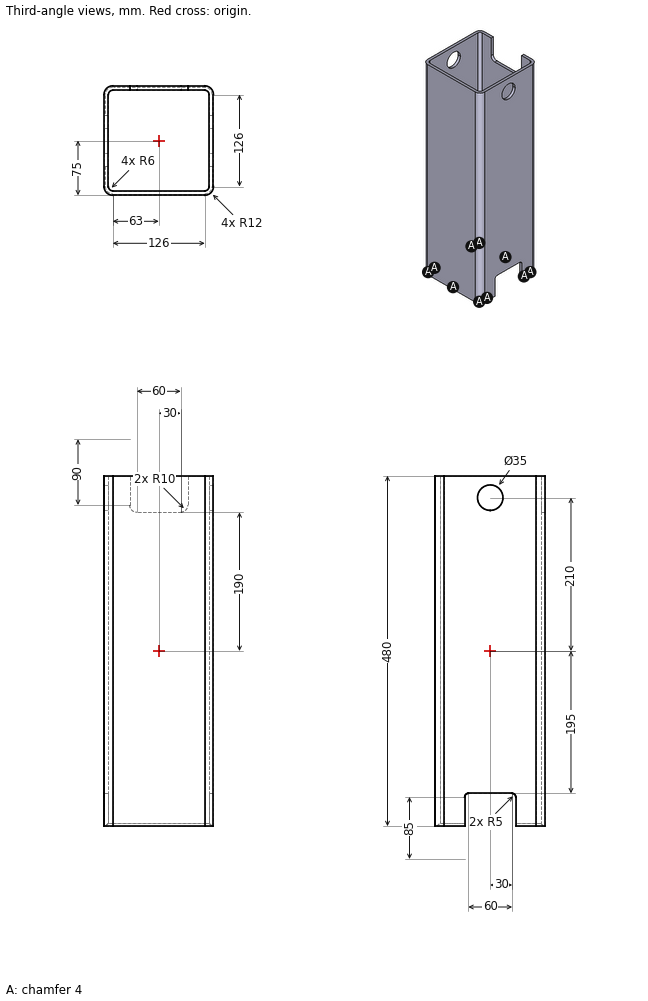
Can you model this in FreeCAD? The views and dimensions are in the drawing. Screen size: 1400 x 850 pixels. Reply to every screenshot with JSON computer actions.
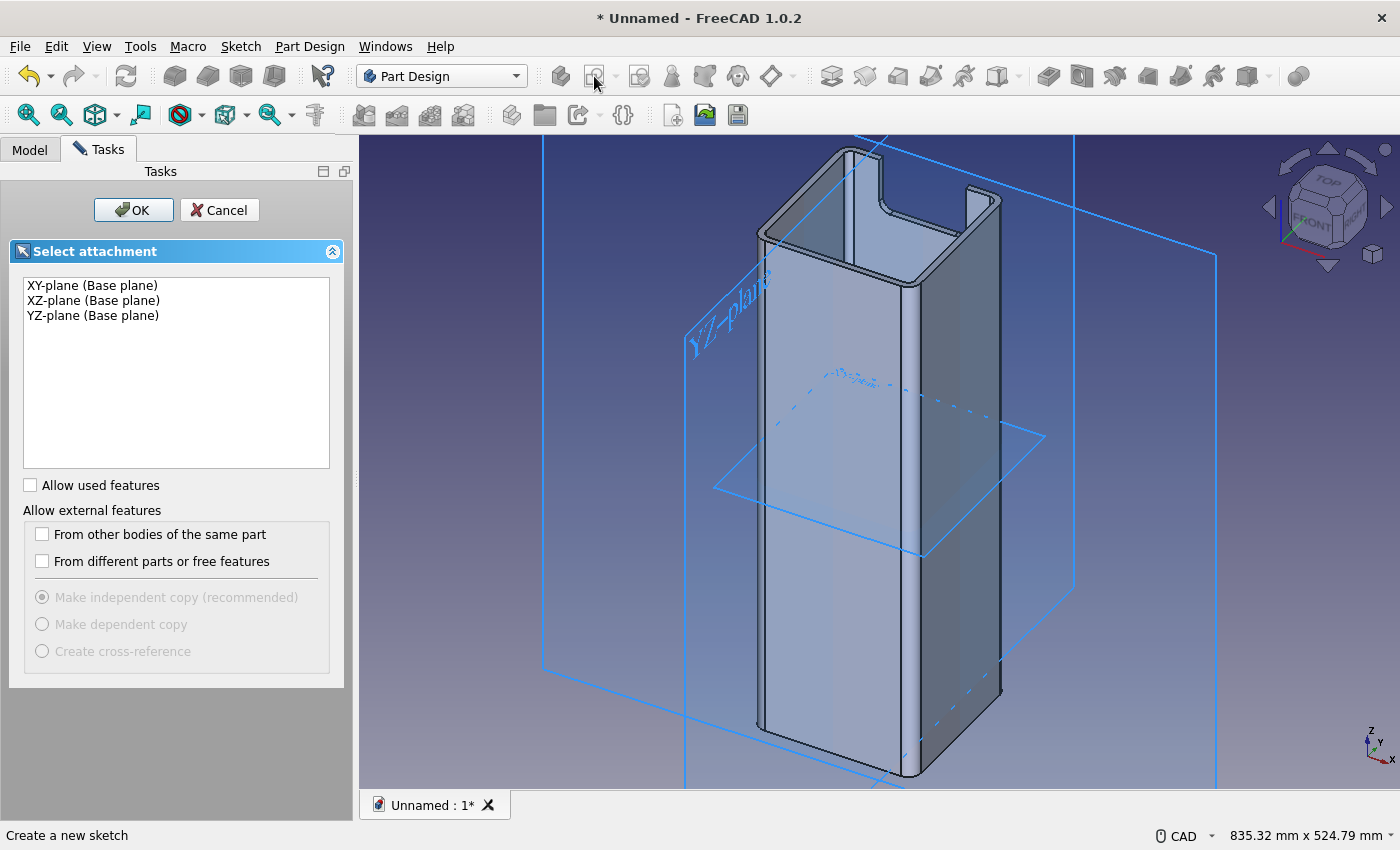
{"action": "left_click", "coordinate": [84, 316]}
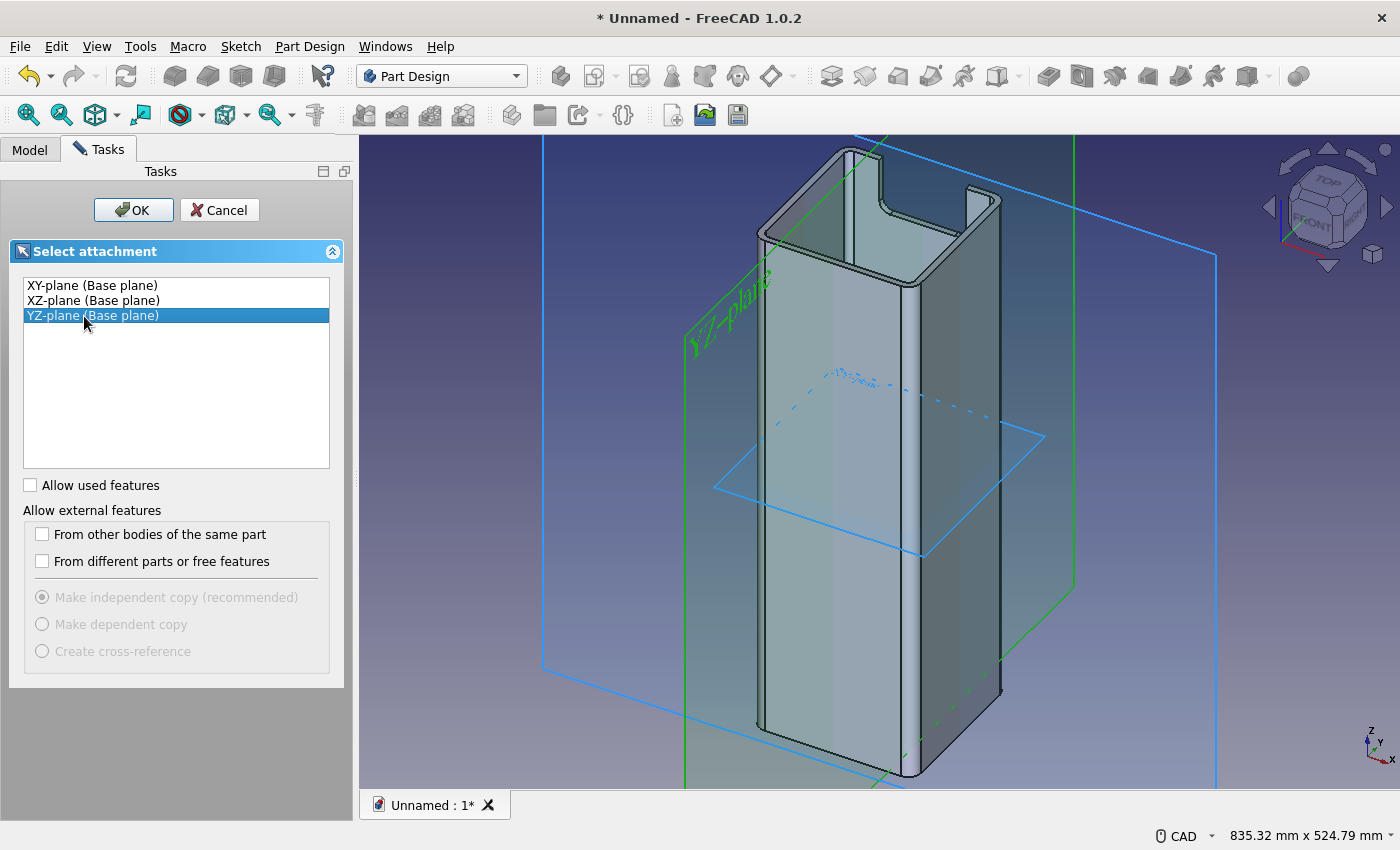
{"action": "left_click", "coordinate": [134, 210]}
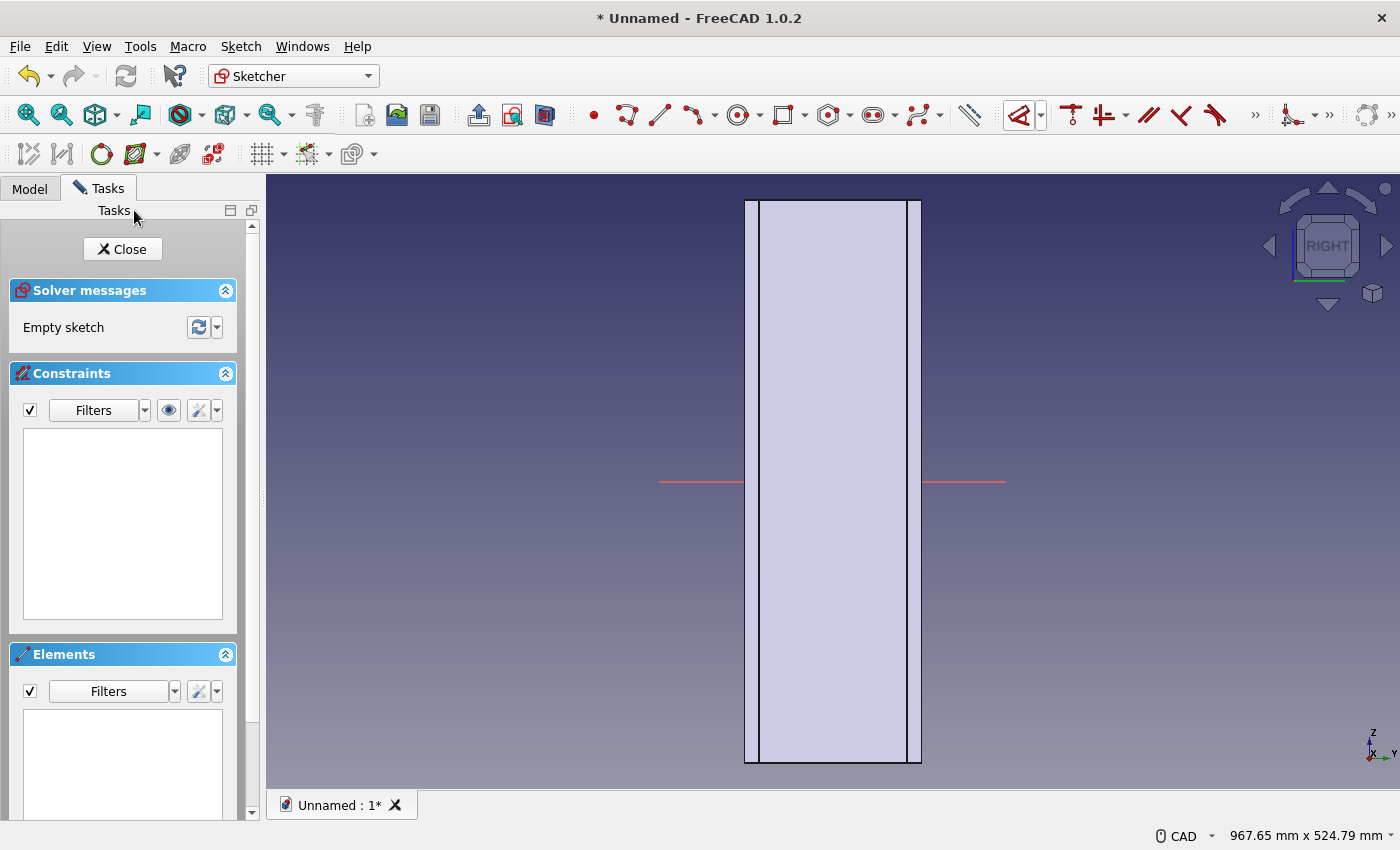
{"action": "left_click", "coordinate": [545, 116]}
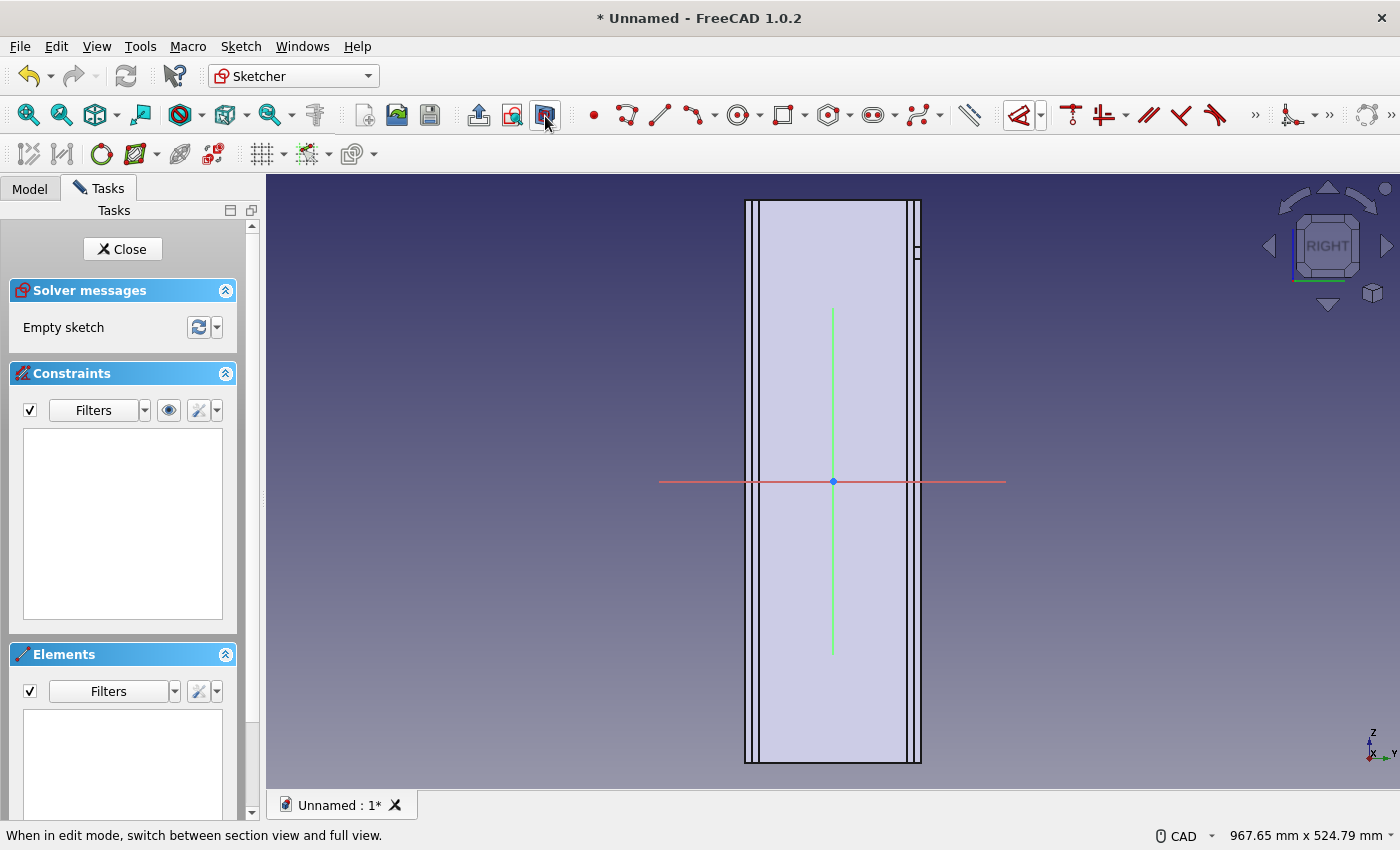
{"action": "scroll", "coordinate": [625, 413], "scroll_direction": "down", "scroll_amount": 2}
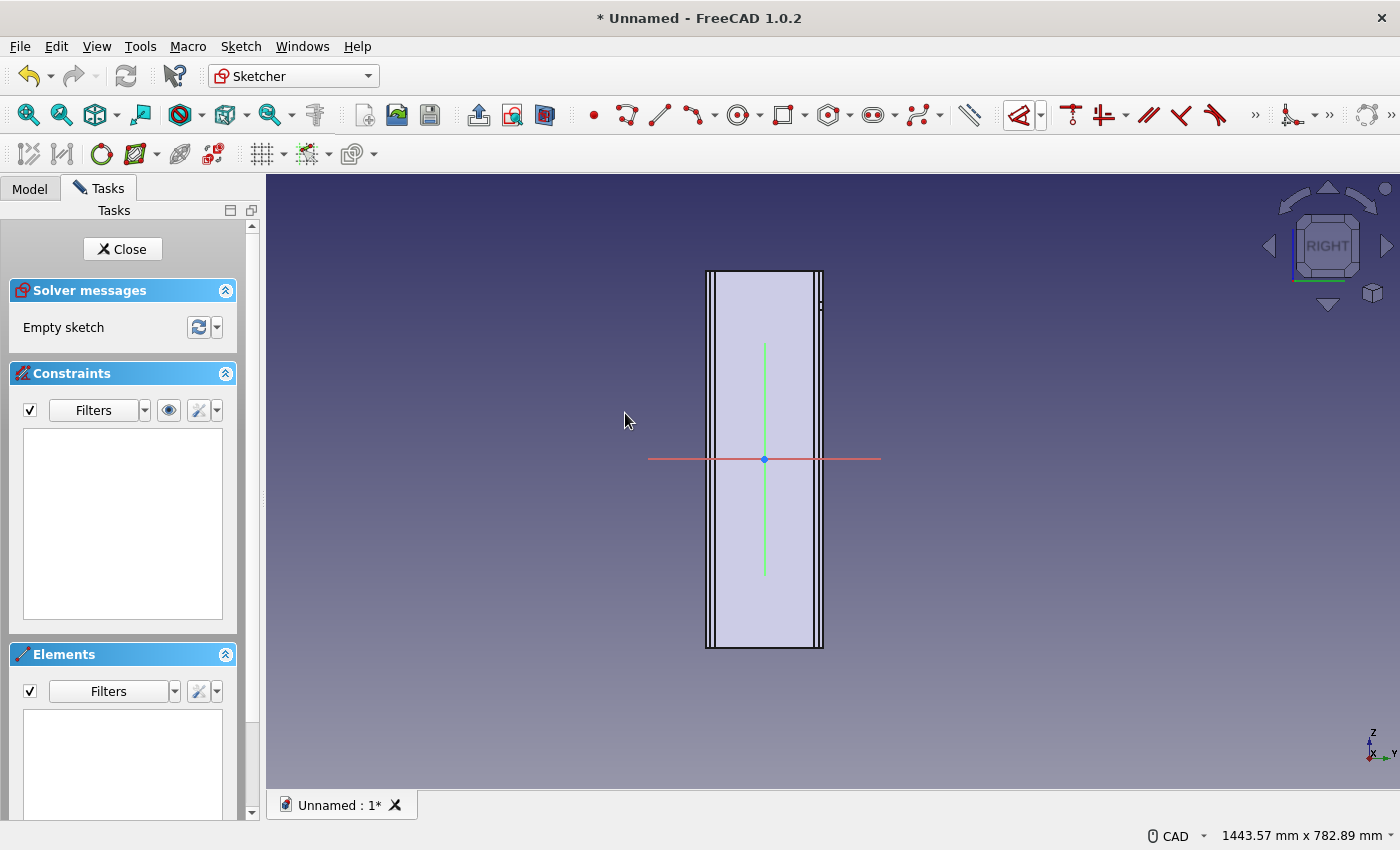
{"action": "left_click", "coordinate": [660, 116]}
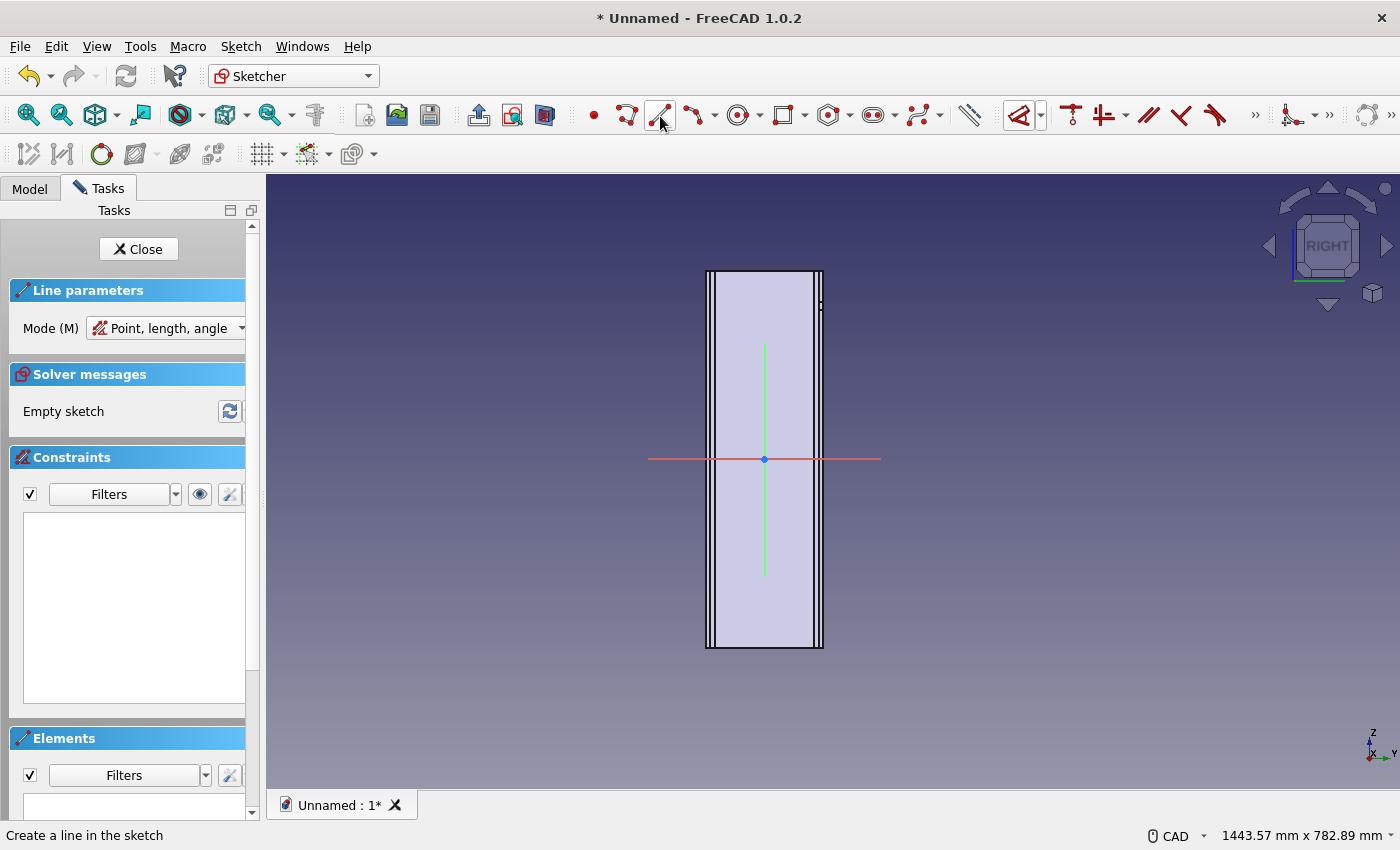
{"action": "left_click", "coordinate": [788, 612]}
{"action": "left_click", "coordinate": [741, 612]}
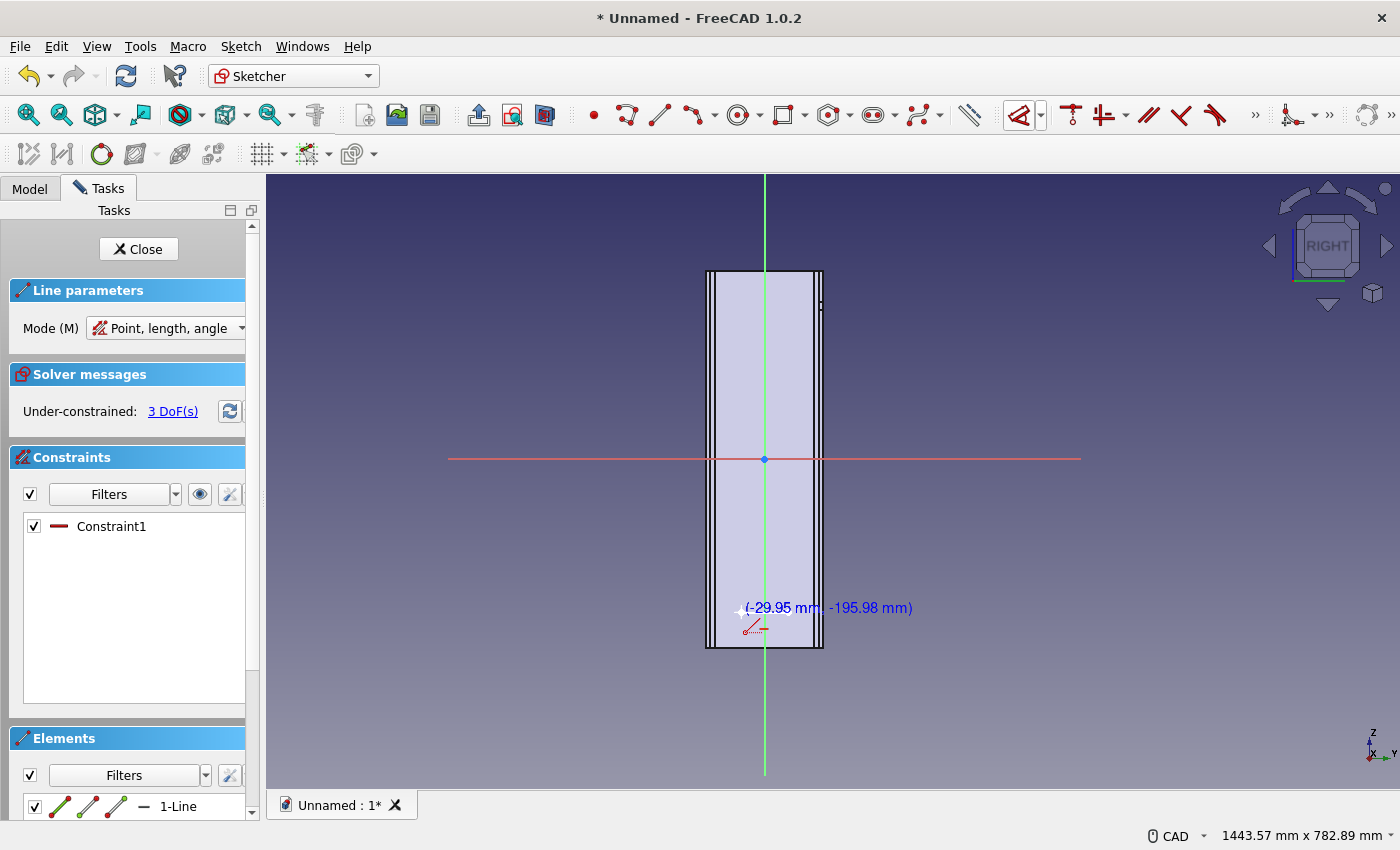
{"action": "left_click", "coordinate": [627, 116]}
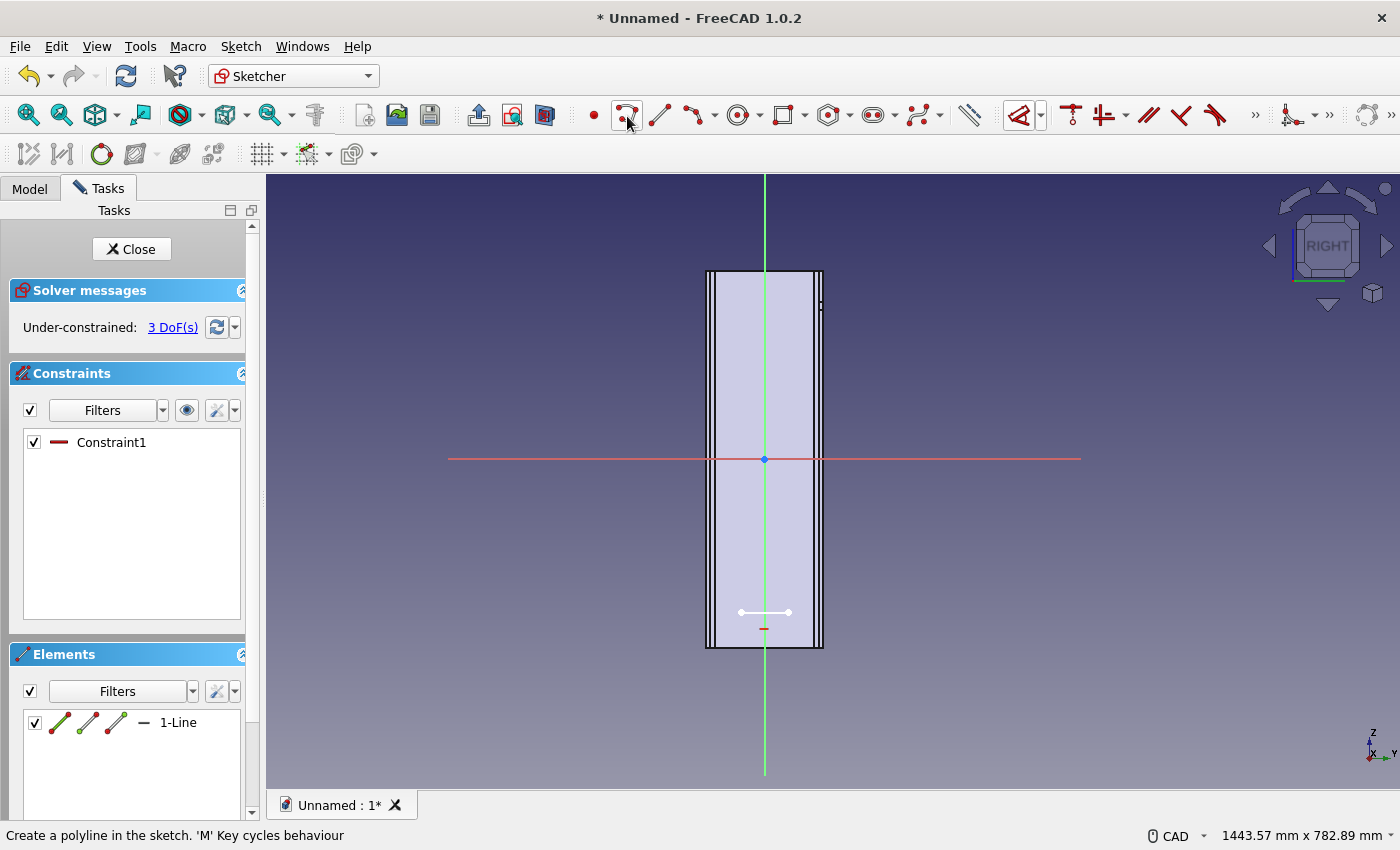
{"action": "scroll", "coordinate": [737, 616], "scroll_direction": "up", "scroll_amount": 6}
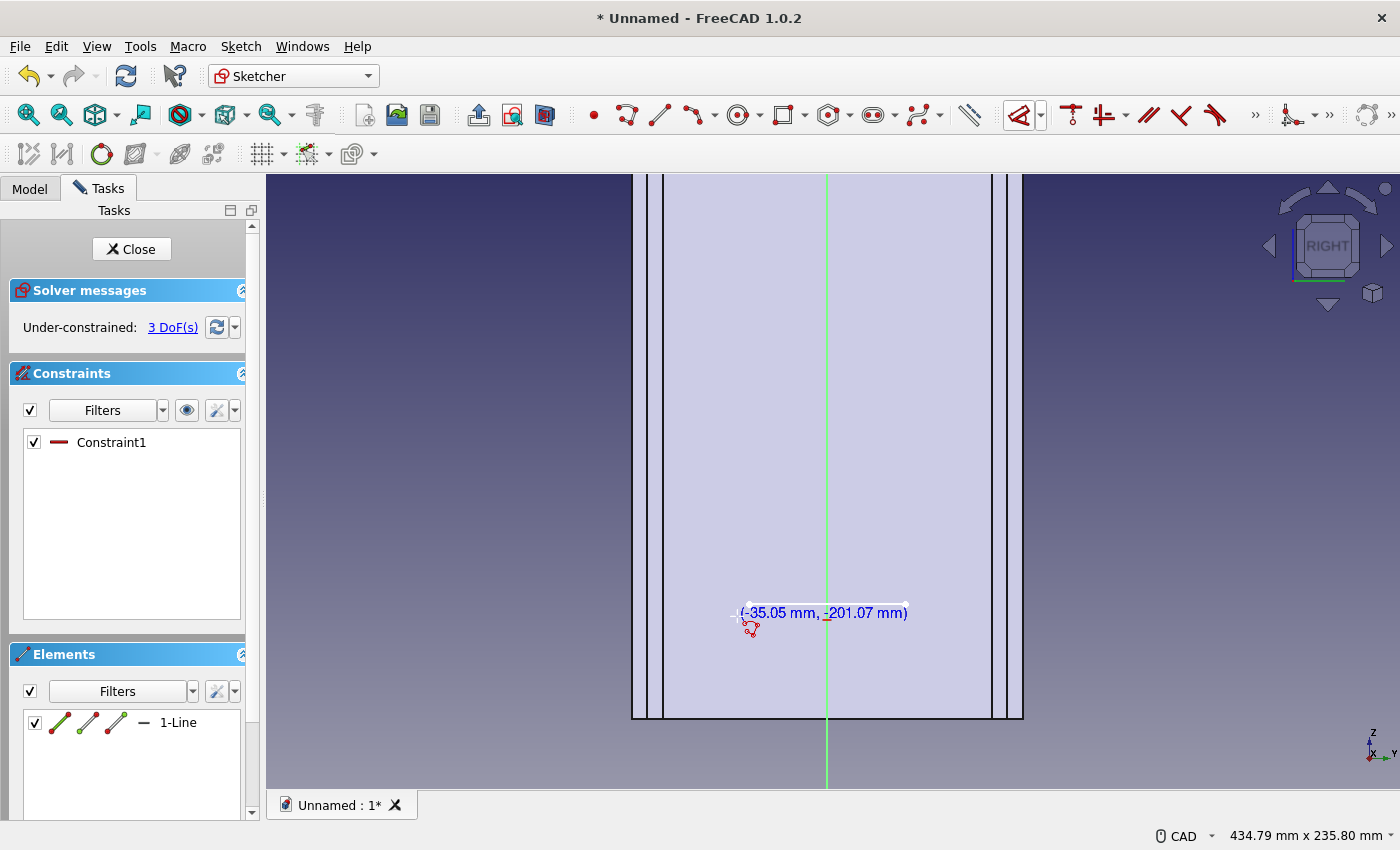
{"action": "left_click", "coordinate": [736, 615]}